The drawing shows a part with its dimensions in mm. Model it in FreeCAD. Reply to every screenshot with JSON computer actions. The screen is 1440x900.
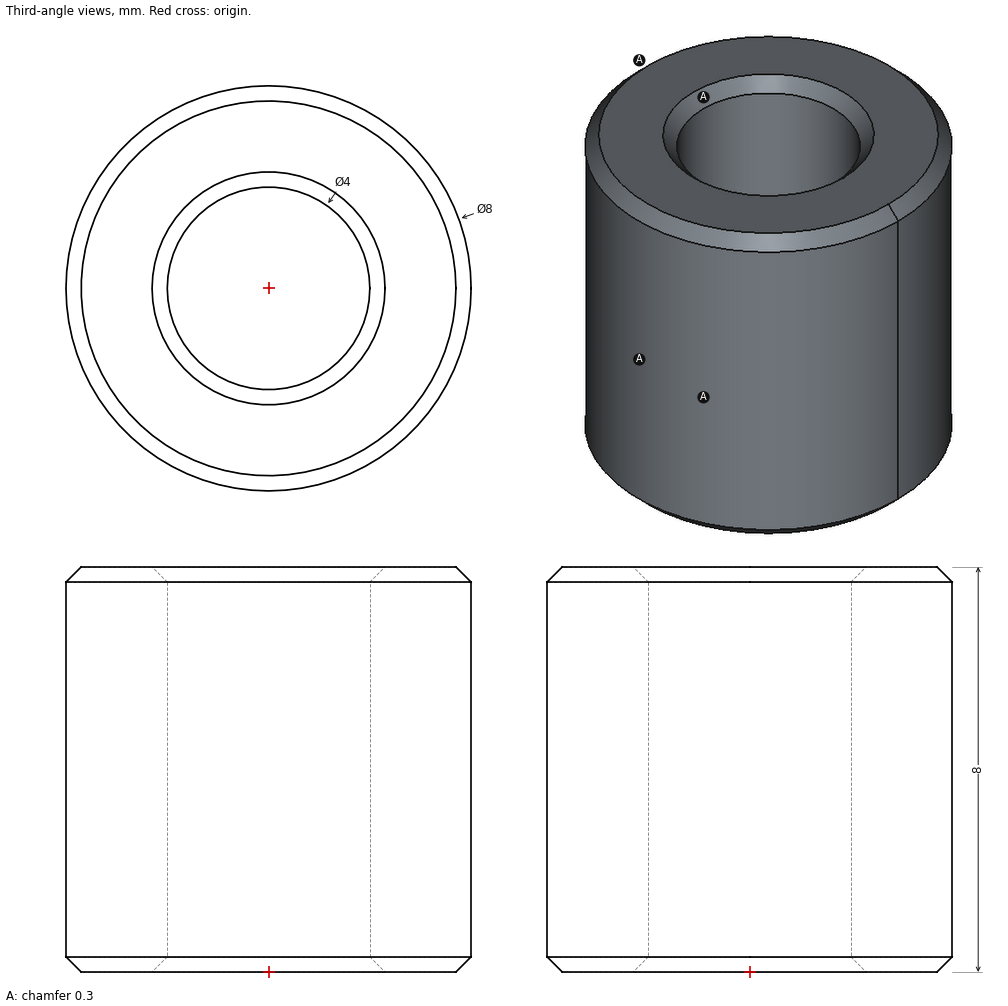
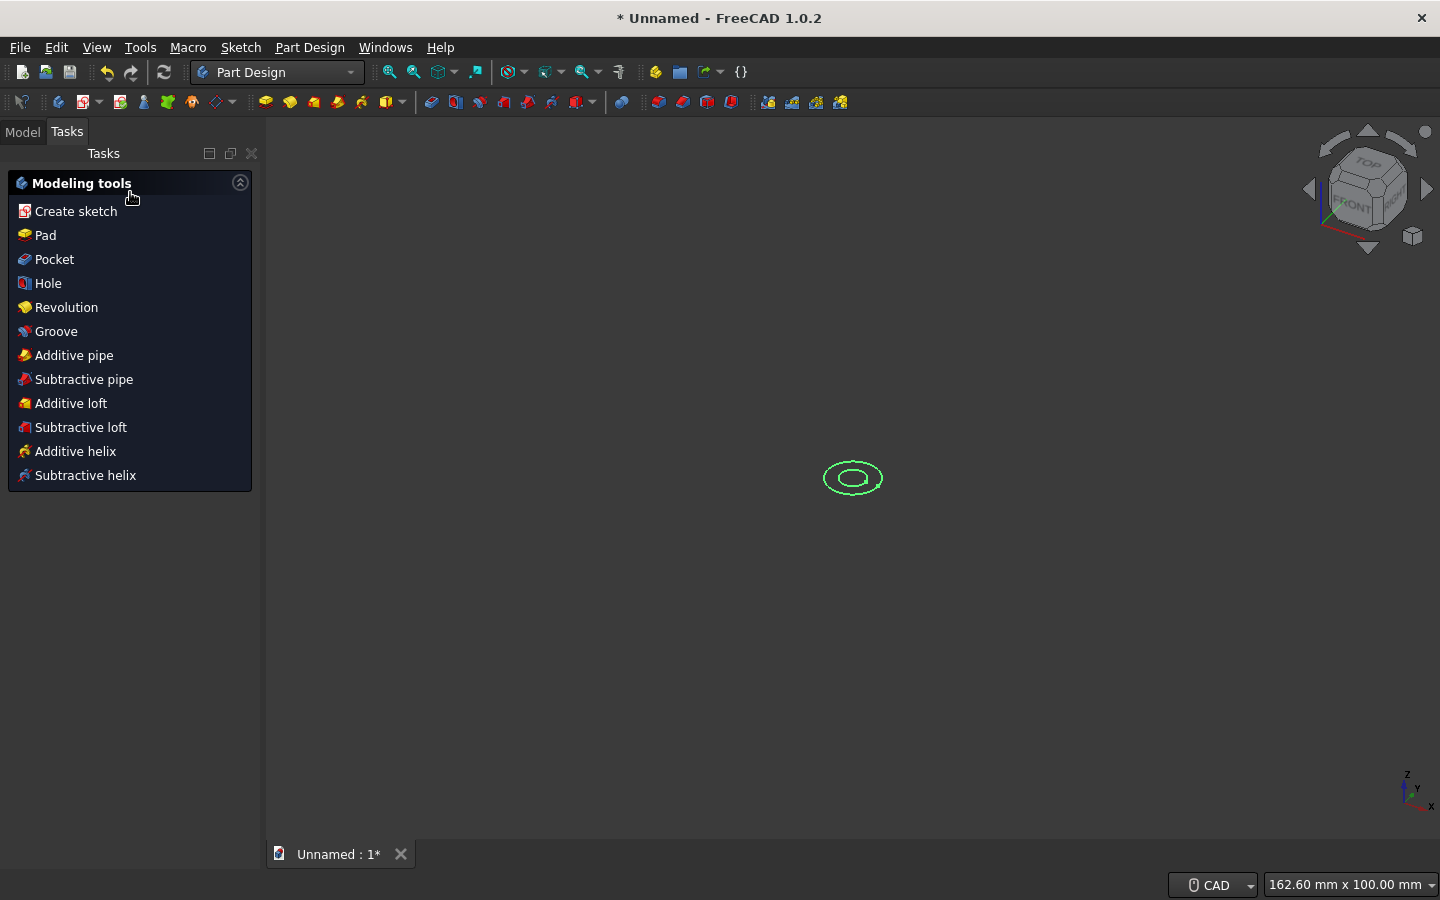
{"action": "left_click", "coordinate": [266, 102]}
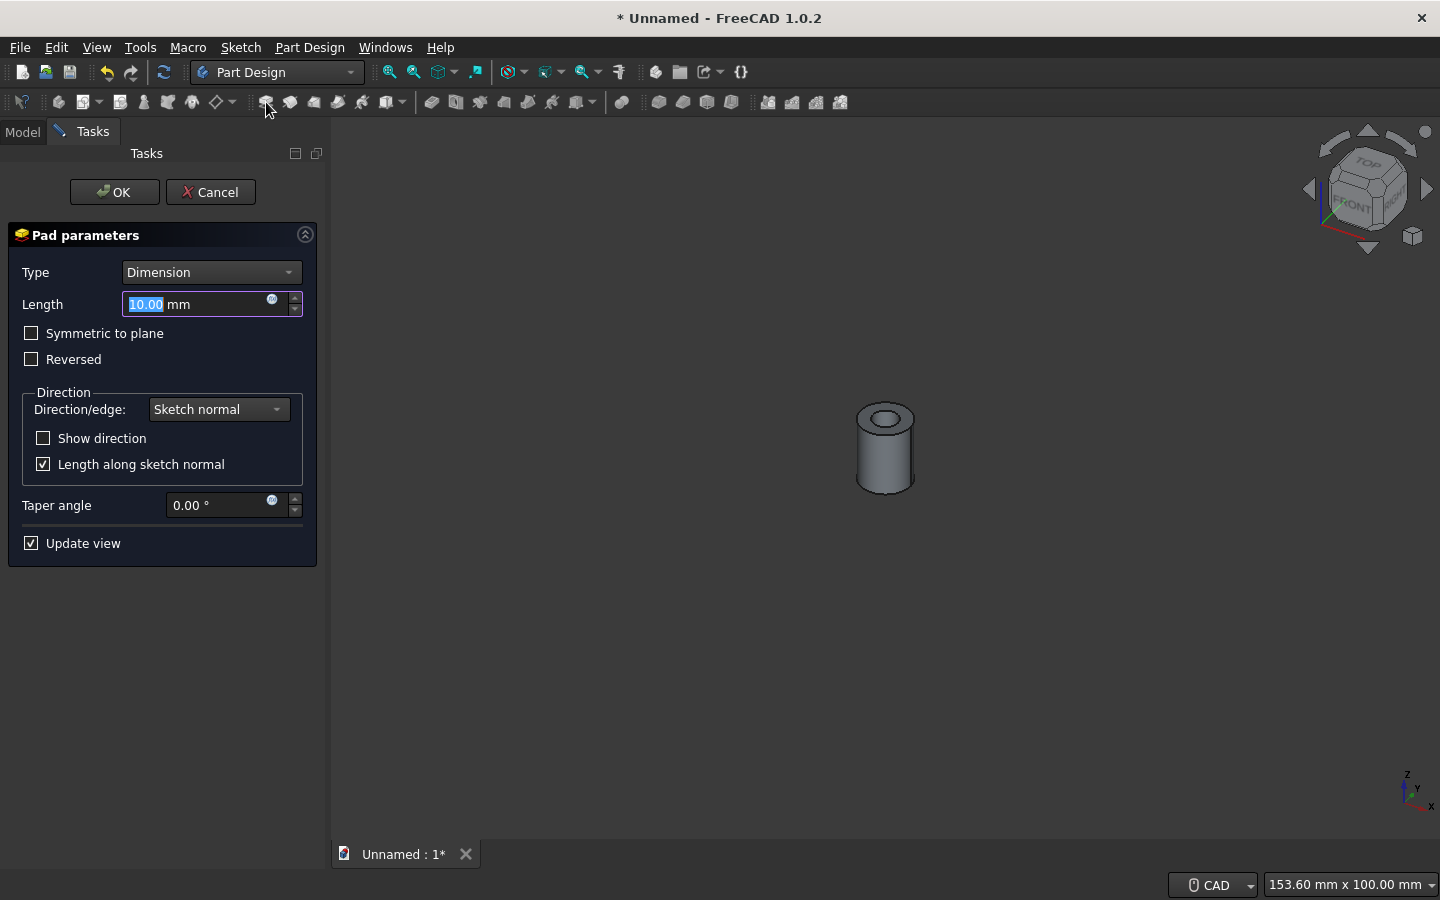
{"action": "type", "text": "8"}
{"action": "key", "text": "Tab"}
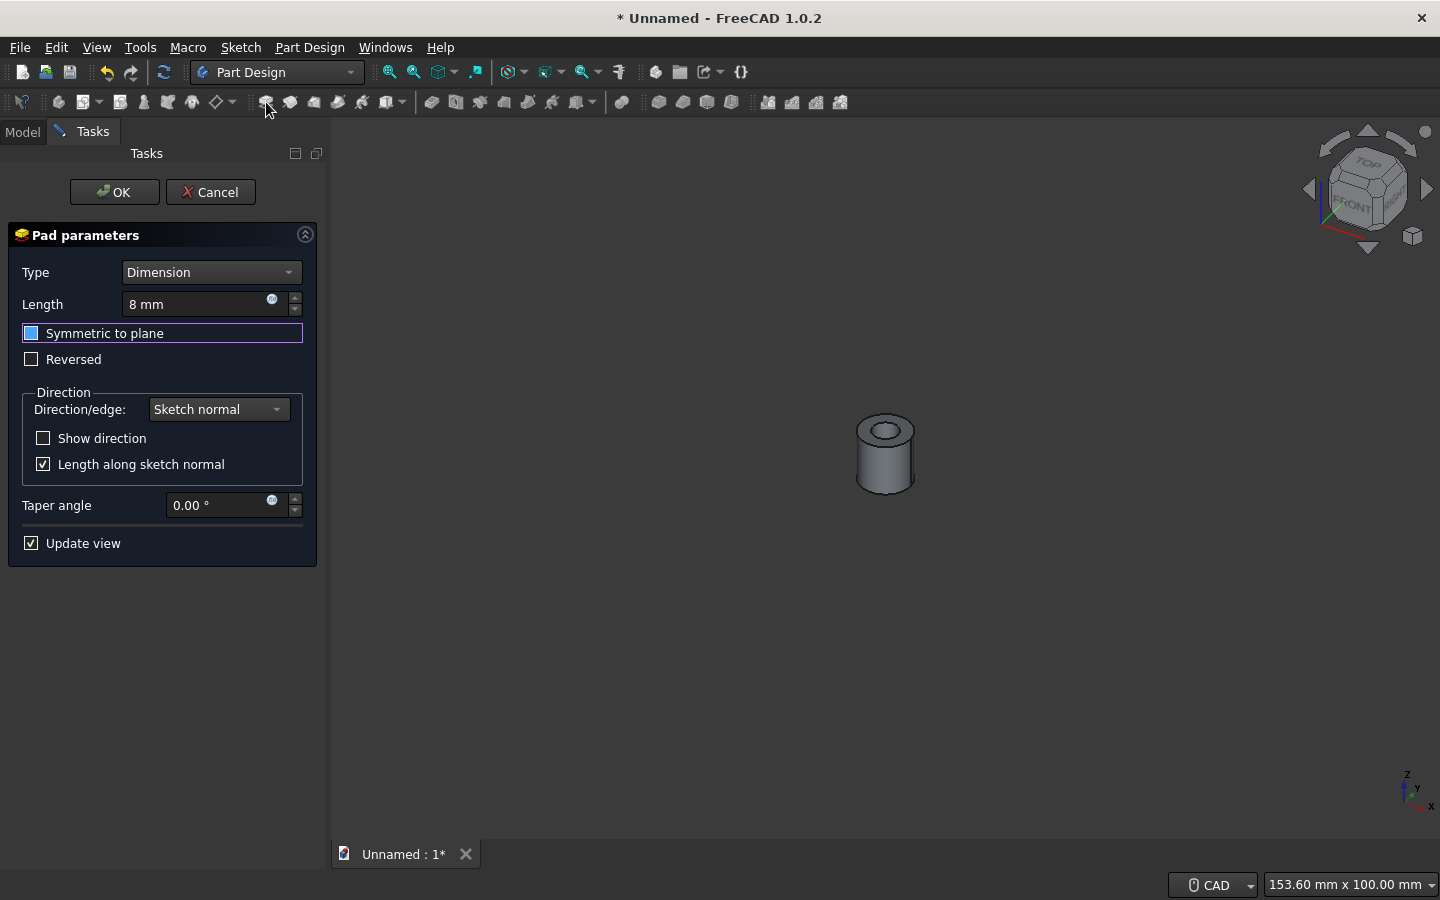
{"action": "left_click", "coordinate": [115, 192]}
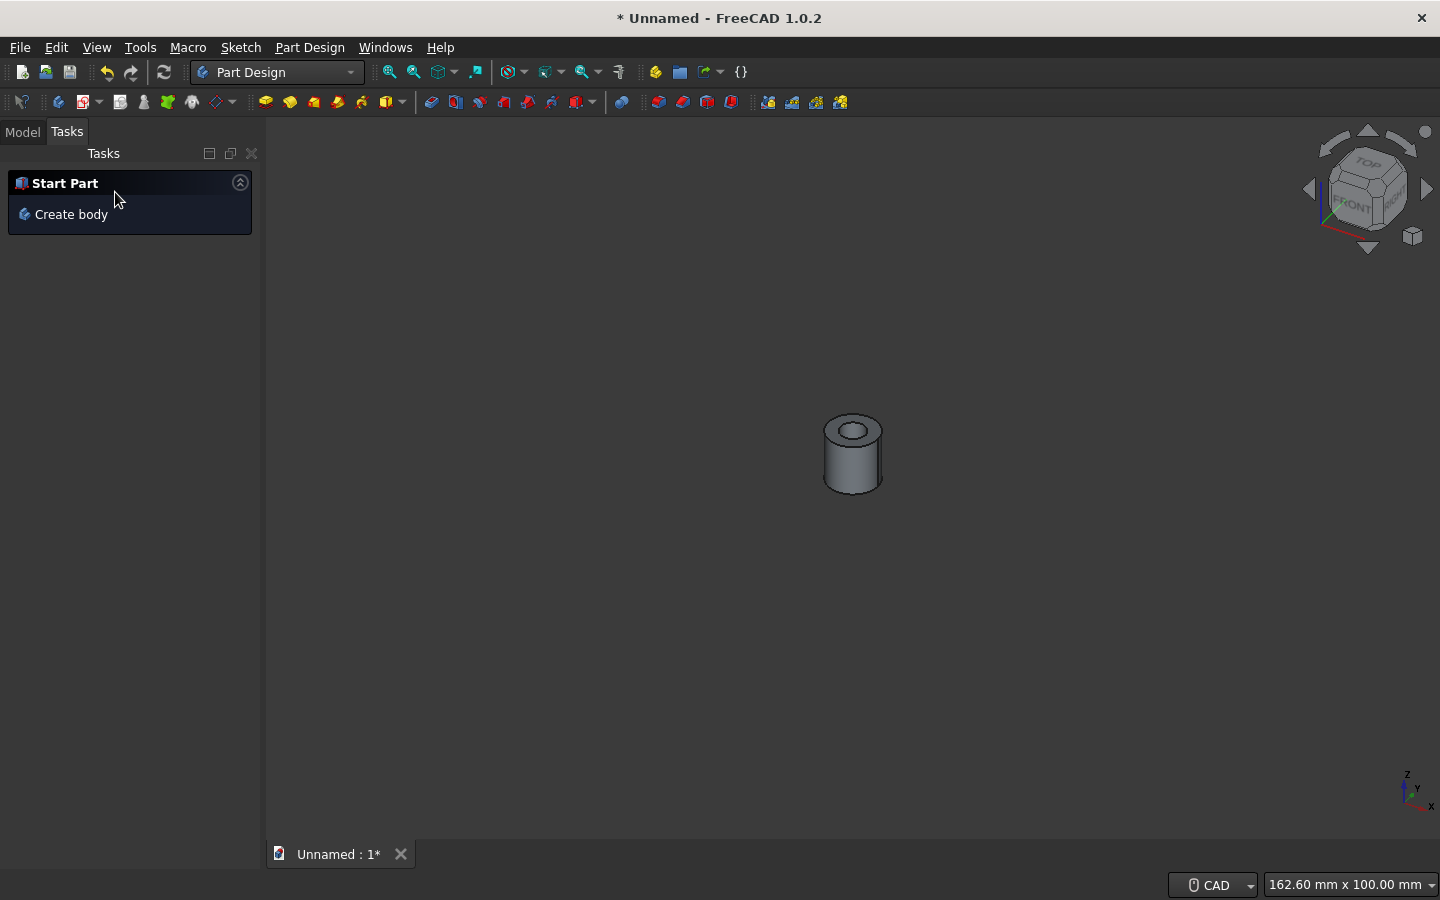
{"action": "key", "text": "v f"}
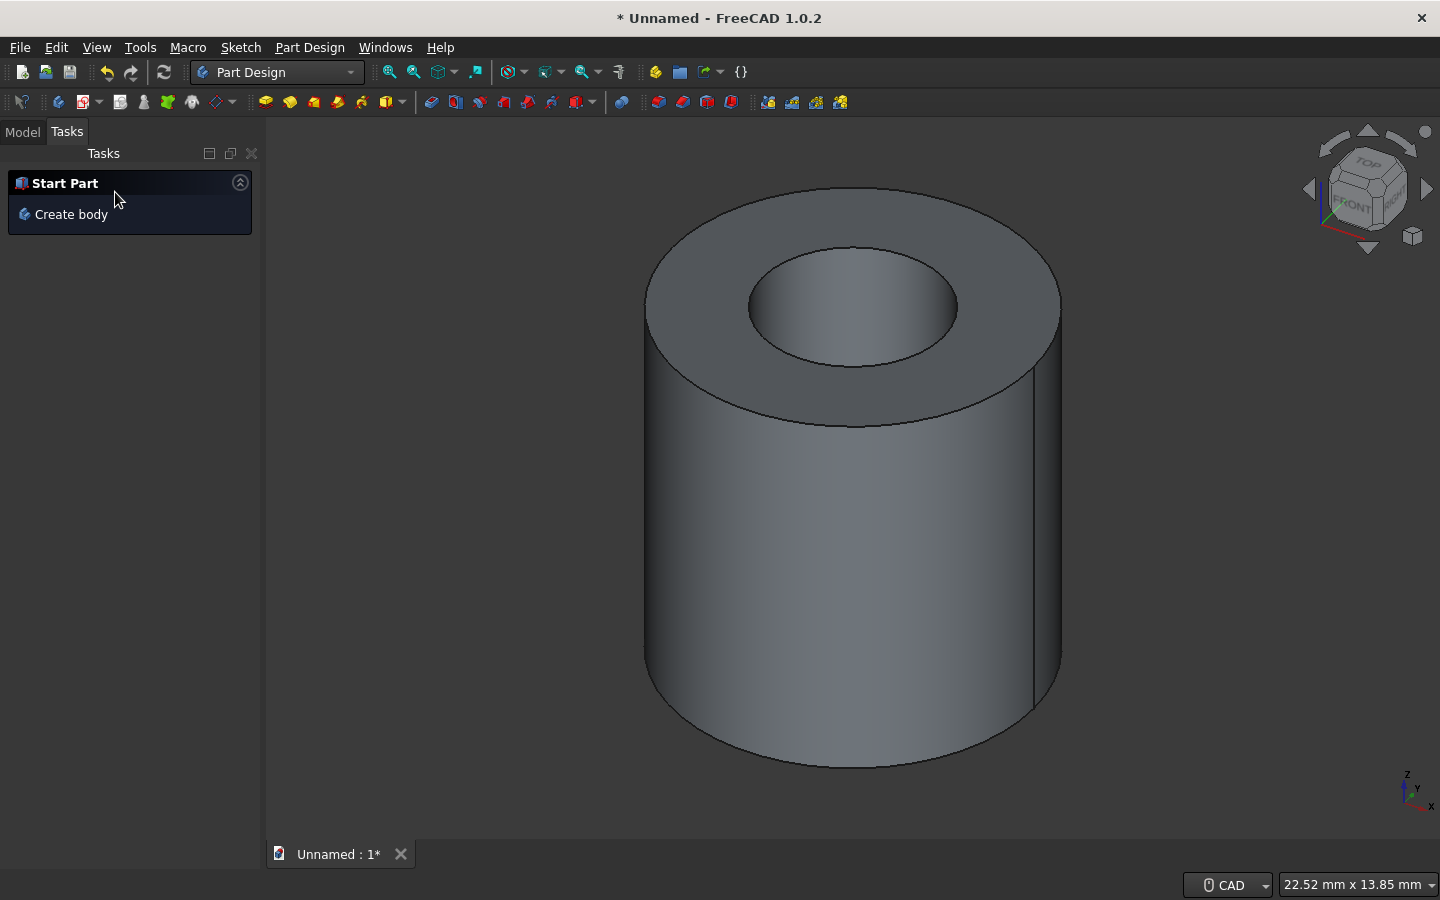
{"action": "left_click", "coordinate": [646, 319]}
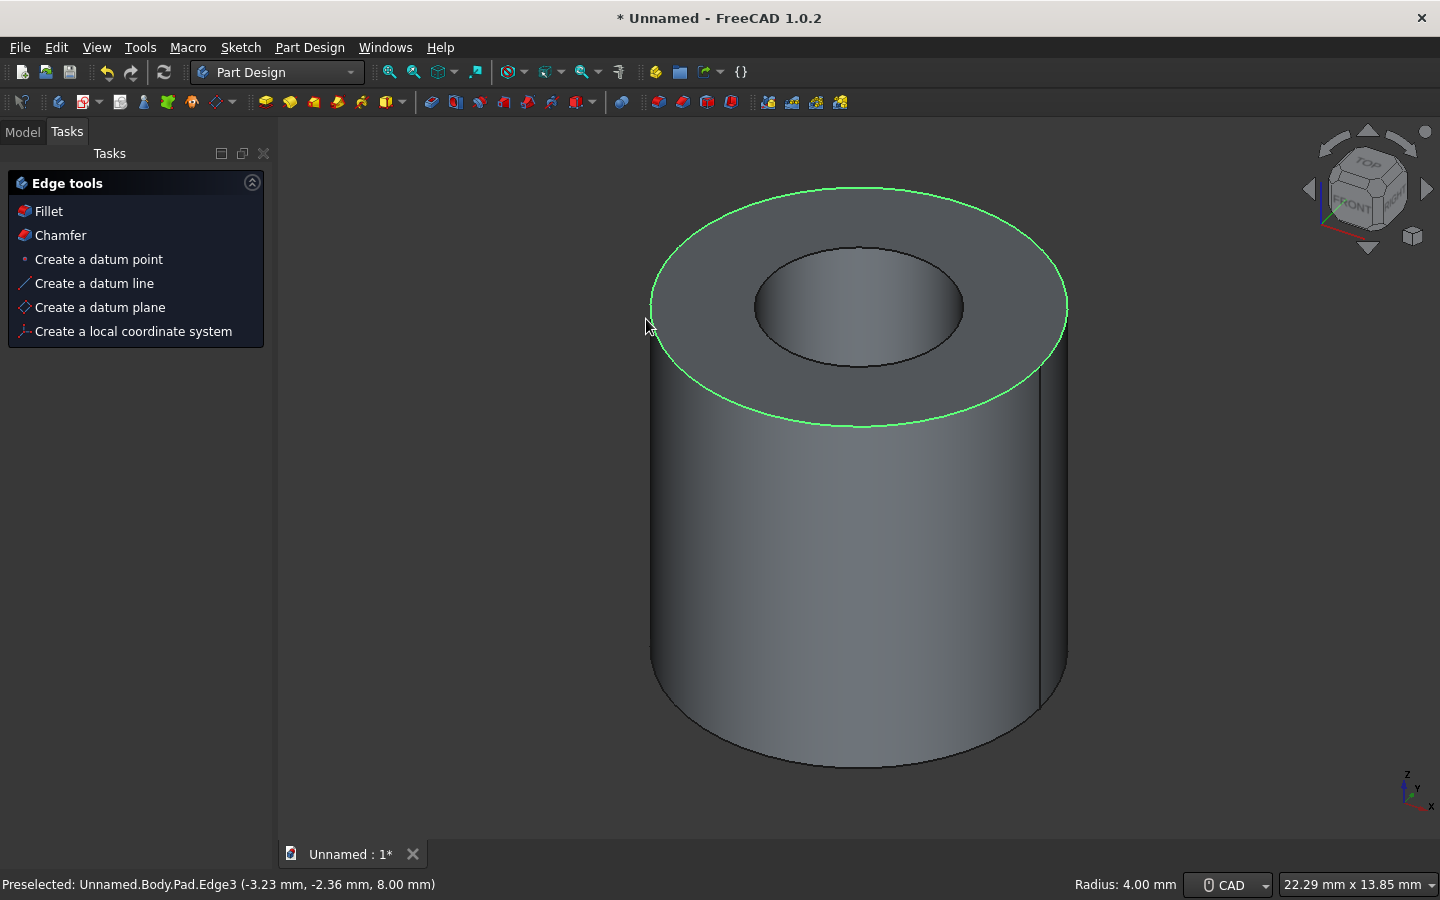
{"action": "left_click", "coordinate": [769, 276], "text": "ctrl"}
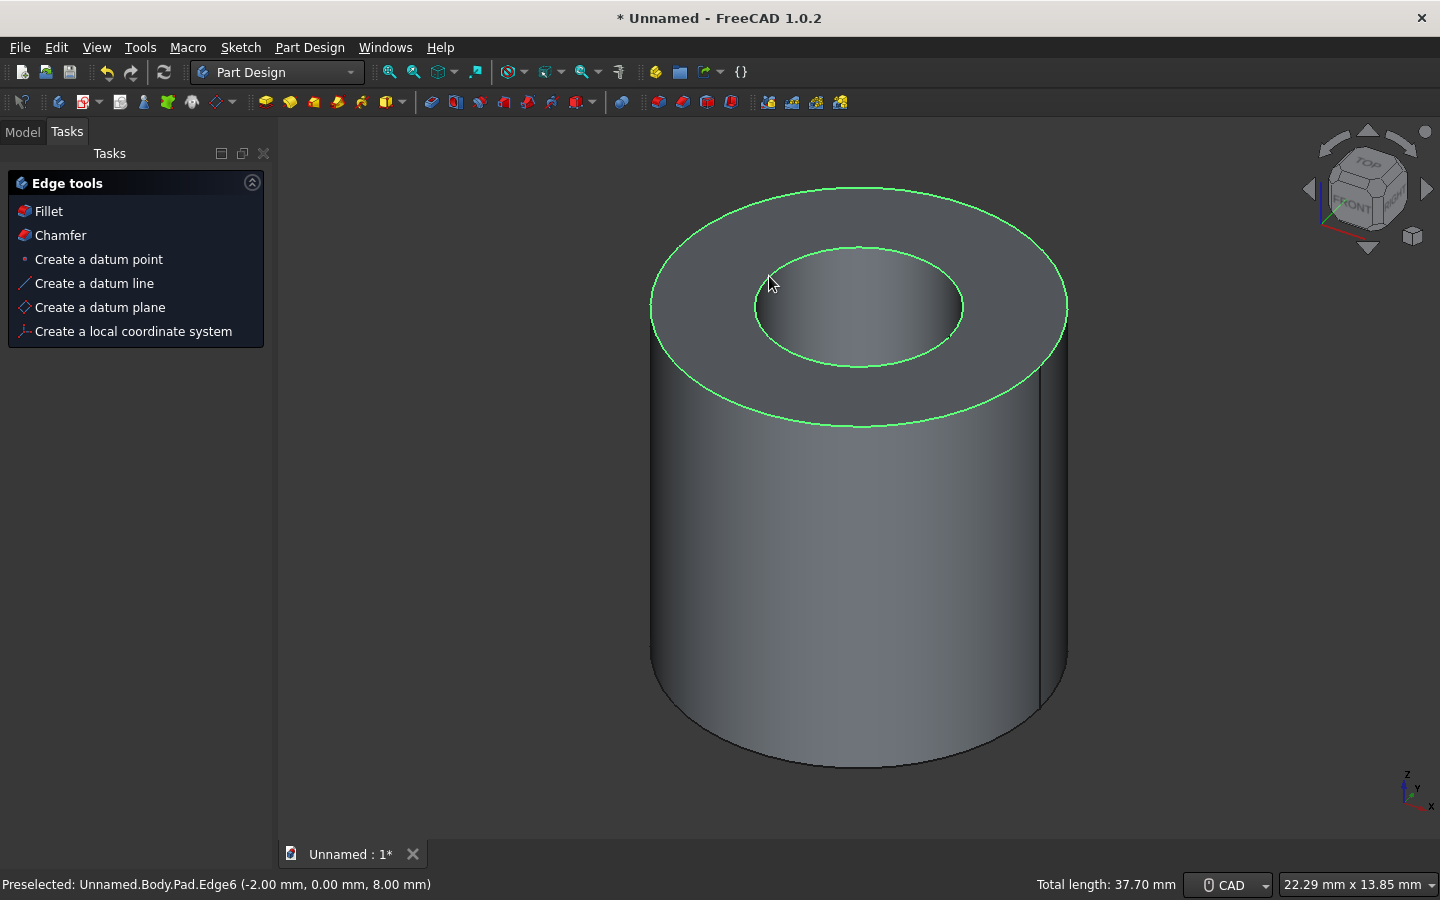
{"action": "key", "text": "0"}